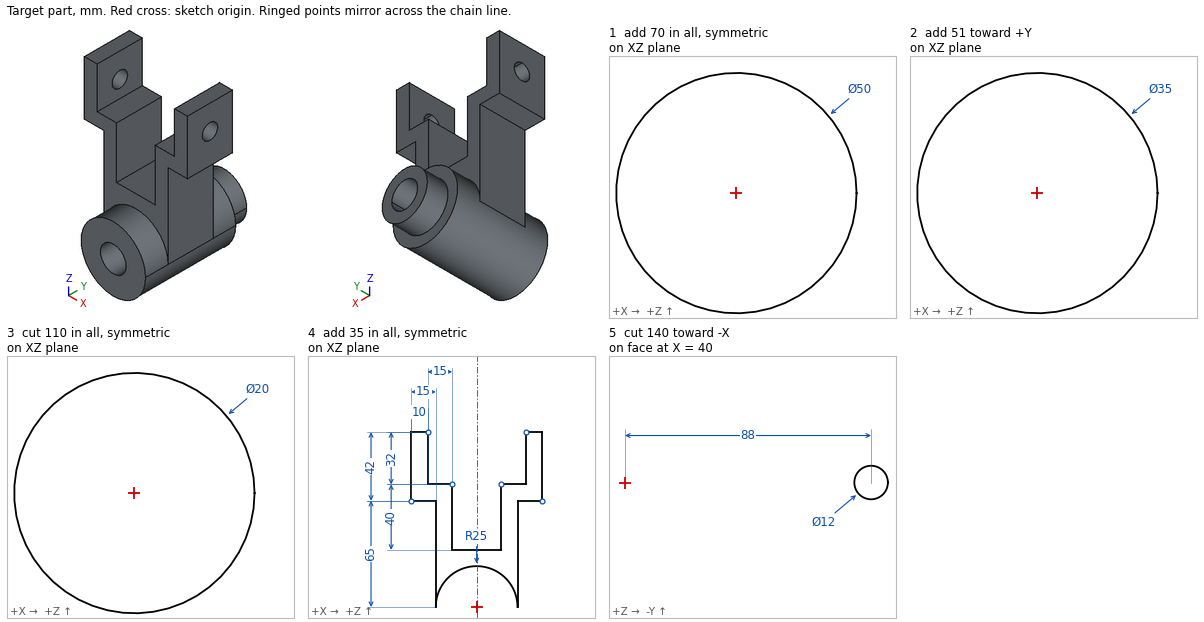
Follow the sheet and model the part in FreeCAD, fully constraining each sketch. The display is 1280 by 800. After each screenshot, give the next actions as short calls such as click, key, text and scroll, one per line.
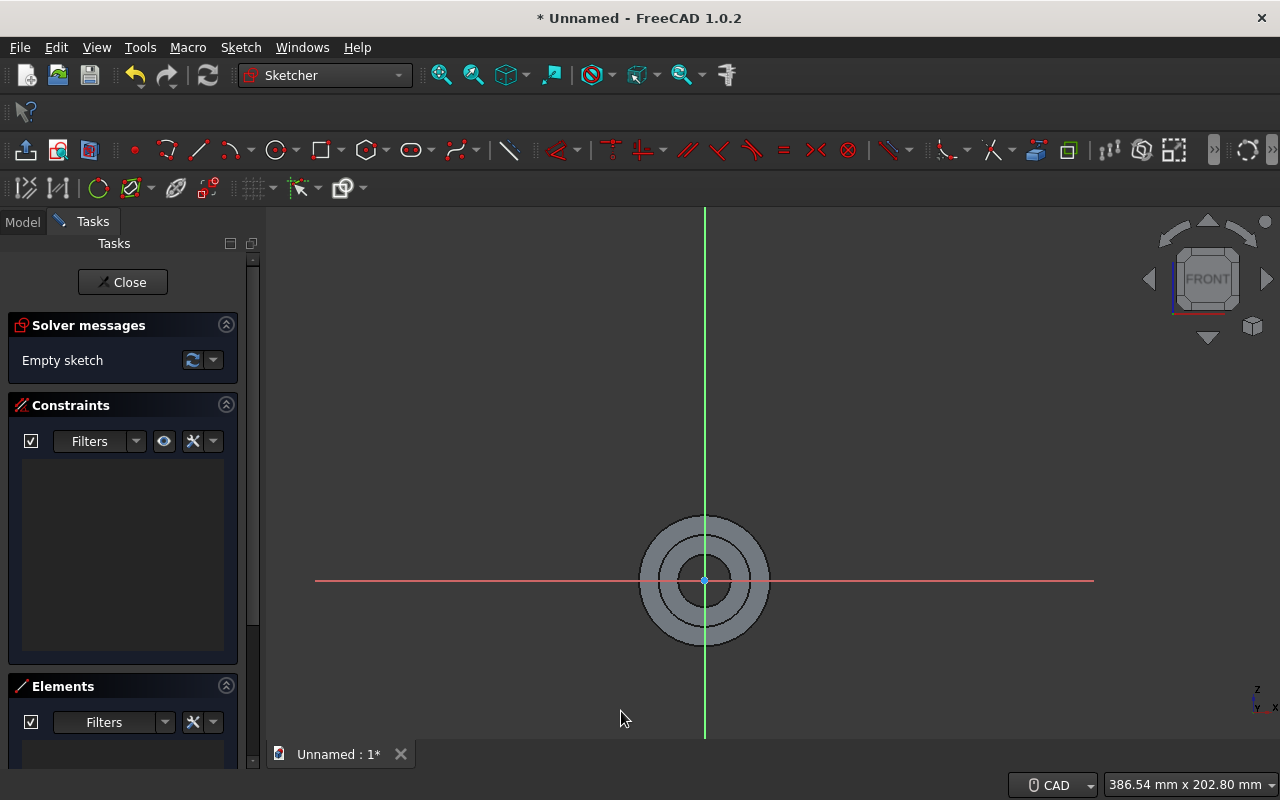
click(168, 150)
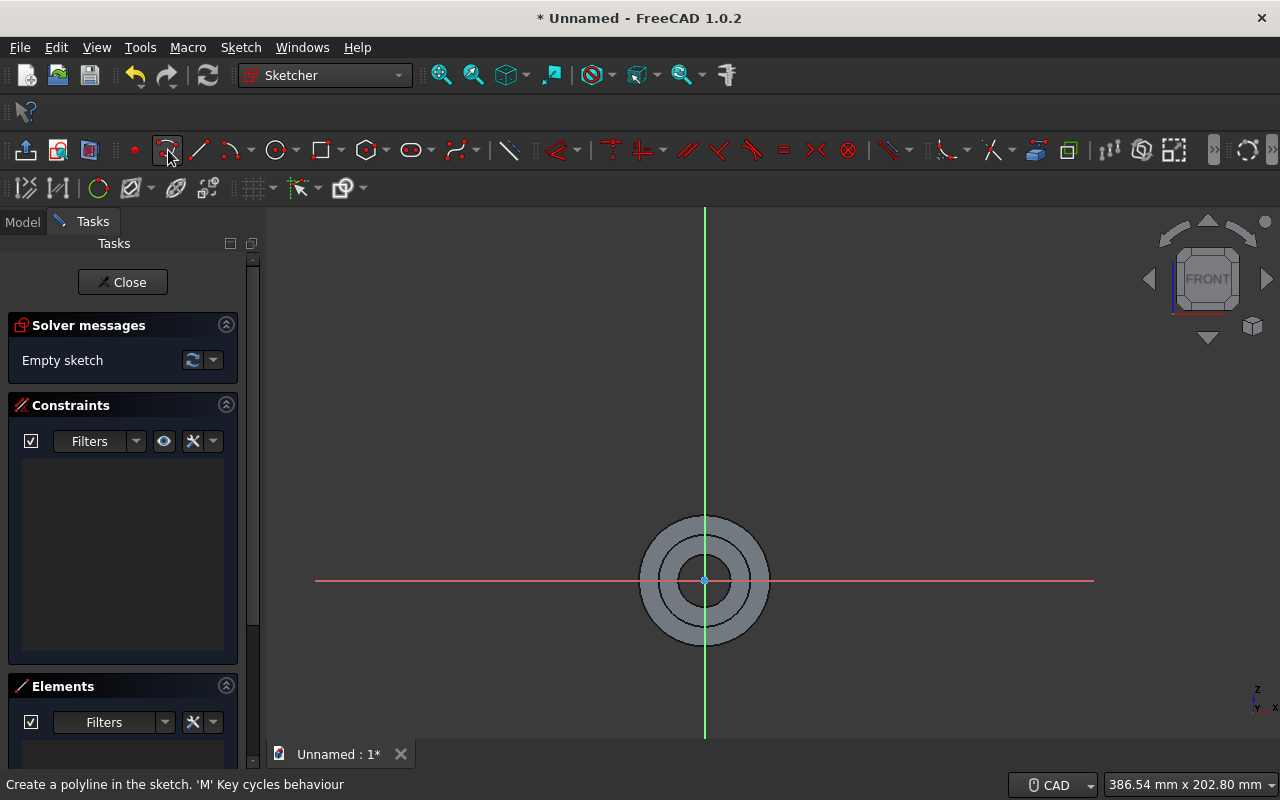
click(639, 581)
click(639, 410)
click(600, 410)
click(600, 300)
click(626, 300)
click(626, 384)
click(665, 384)
click(665, 489)
click(744, 489)
click(744, 384)
click(783, 384)
click(783, 300)
click(809, 300)
click(809, 410)
click(770, 410)
click(770, 581)
right_click(770, 581)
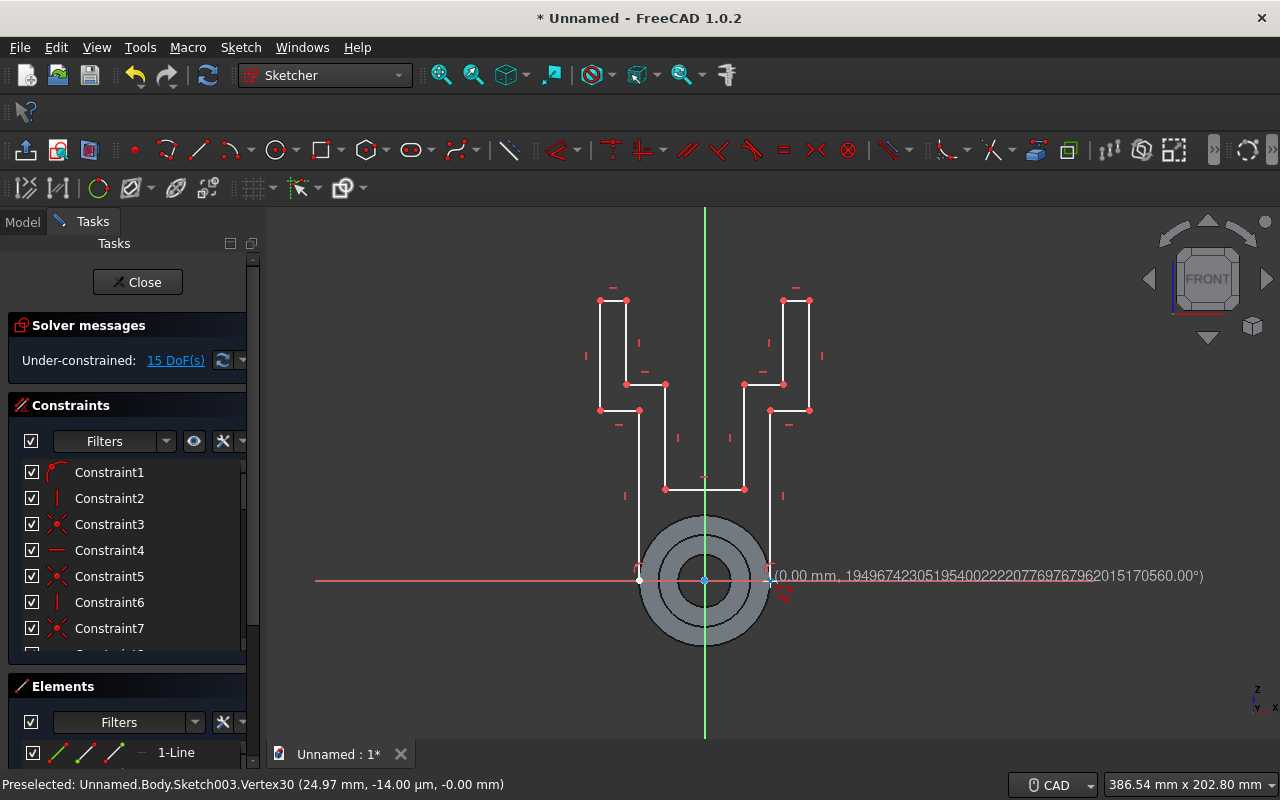
click(254, 150)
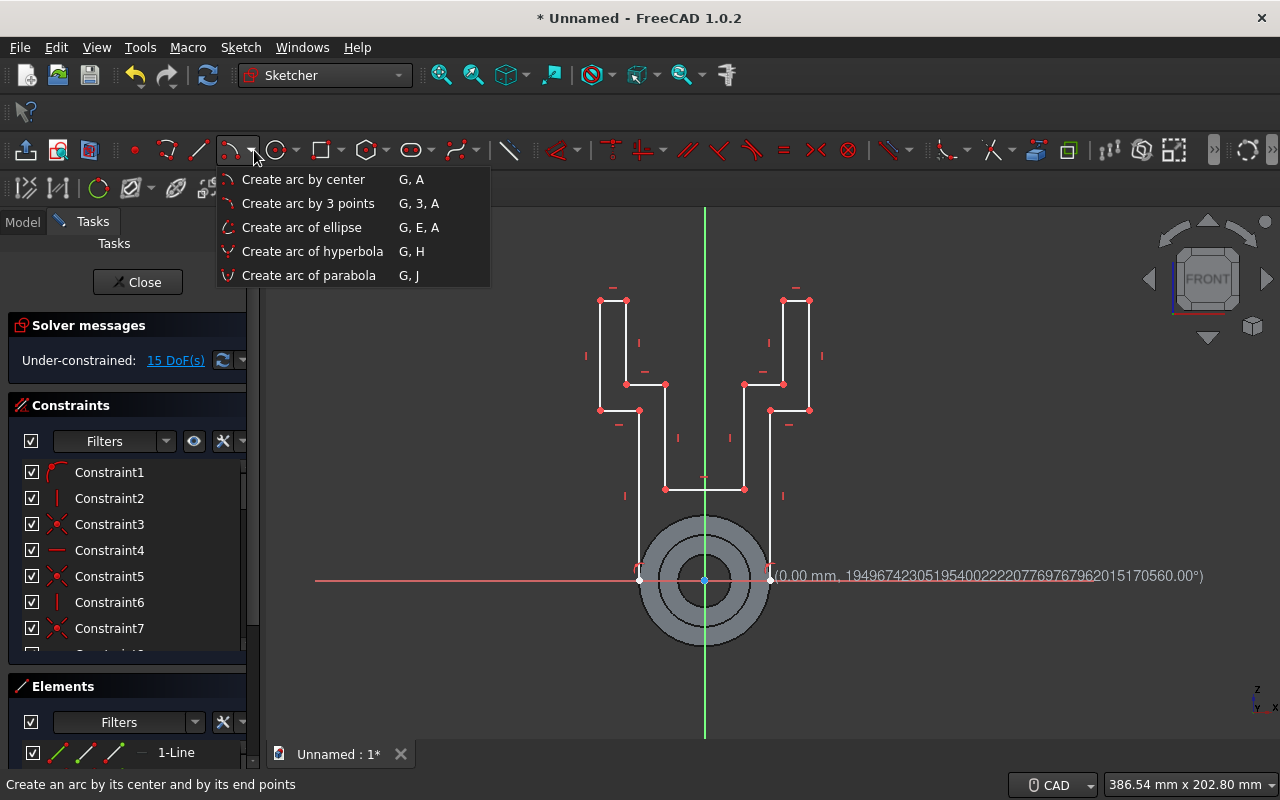
click(354, 203)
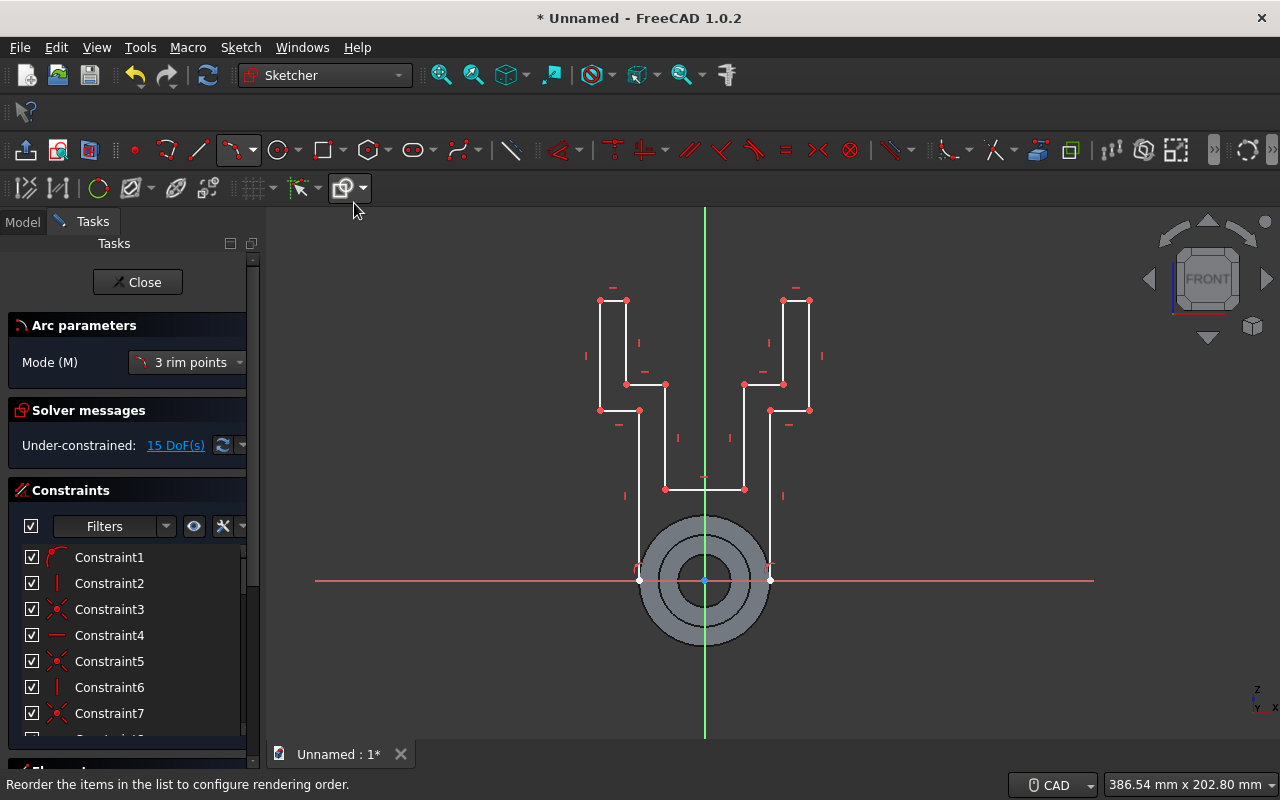
click(770, 581)
click(639, 581)
click(725, 518)
key(Escape)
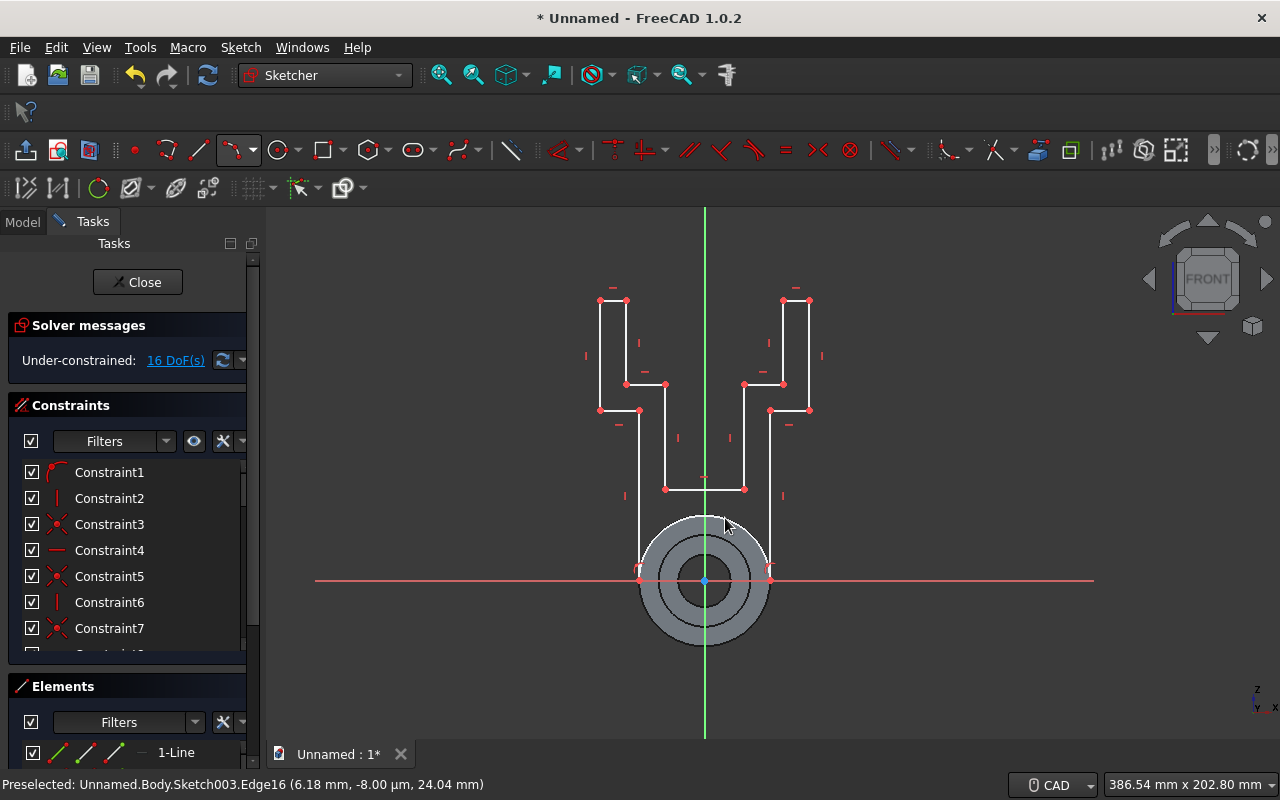
click(639, 530)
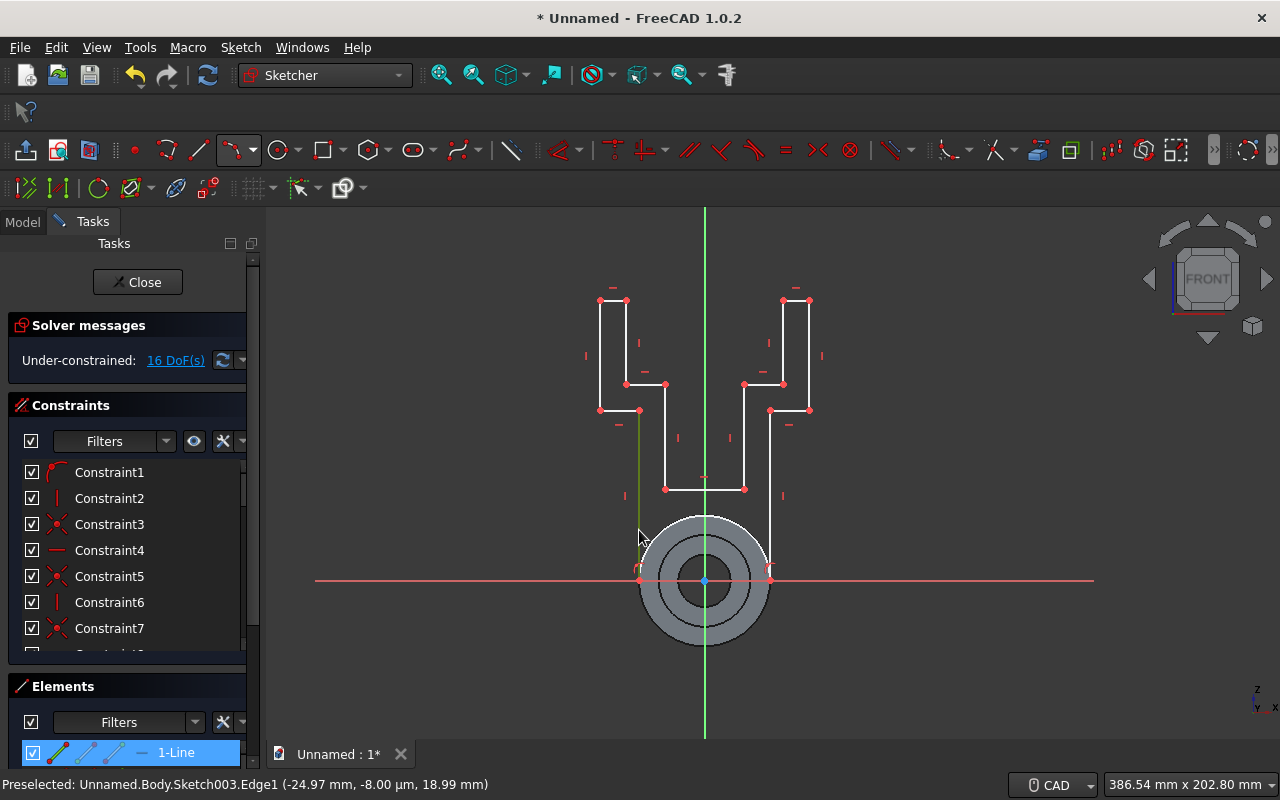
click(743, 528)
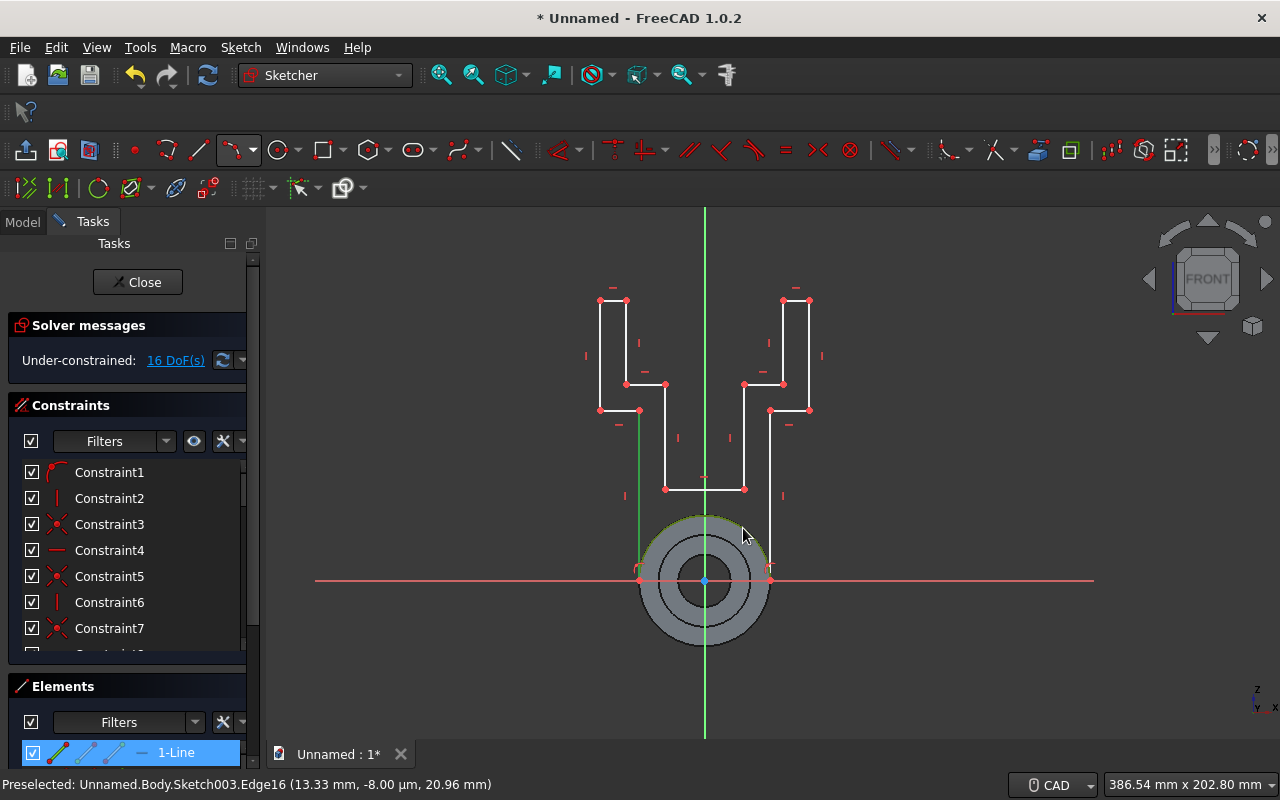
click(754, 150)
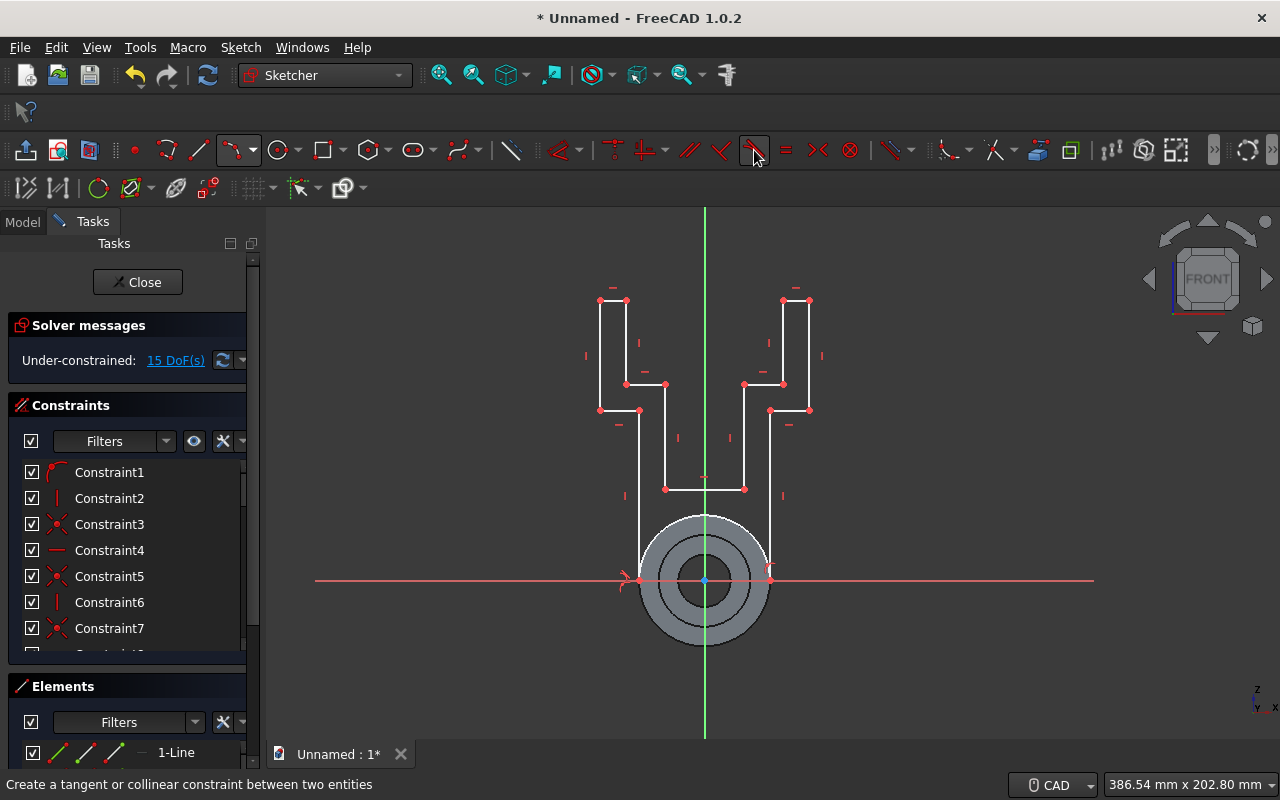
click(705, 581)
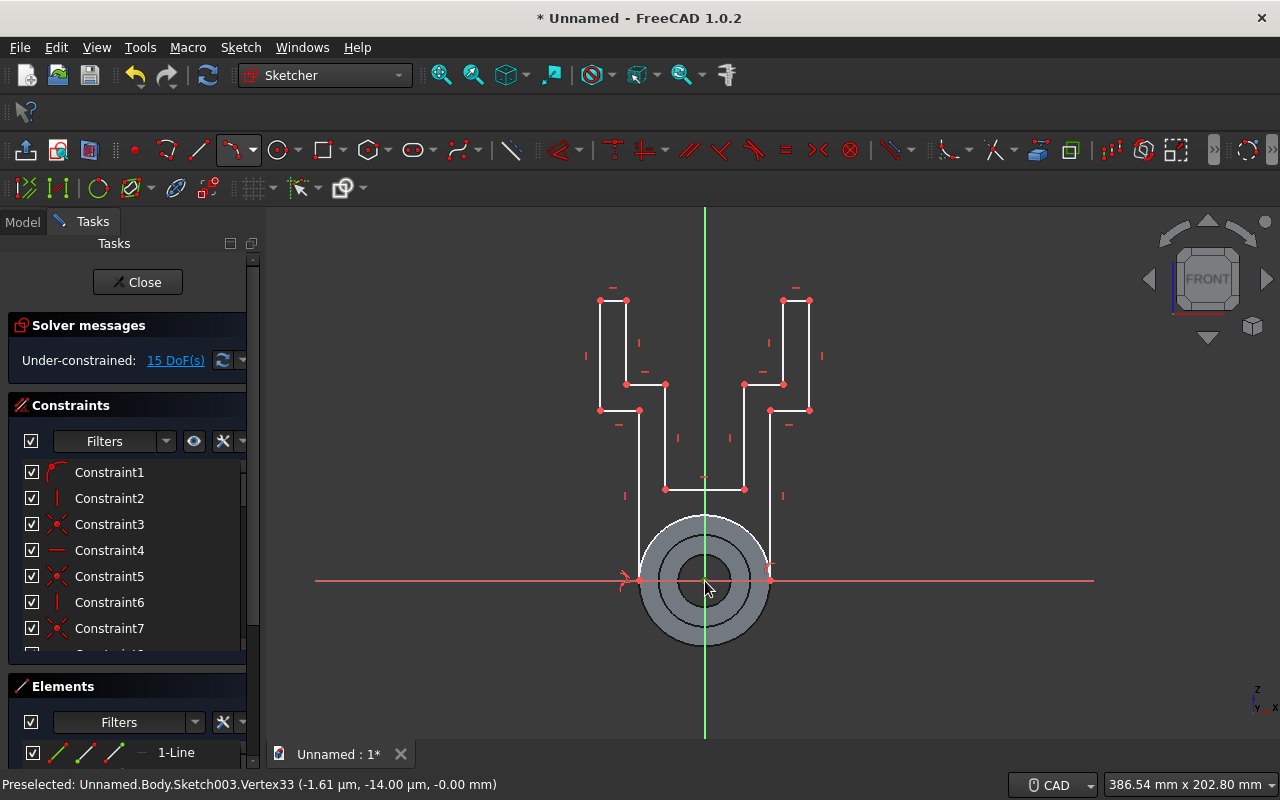
click(705, 677)